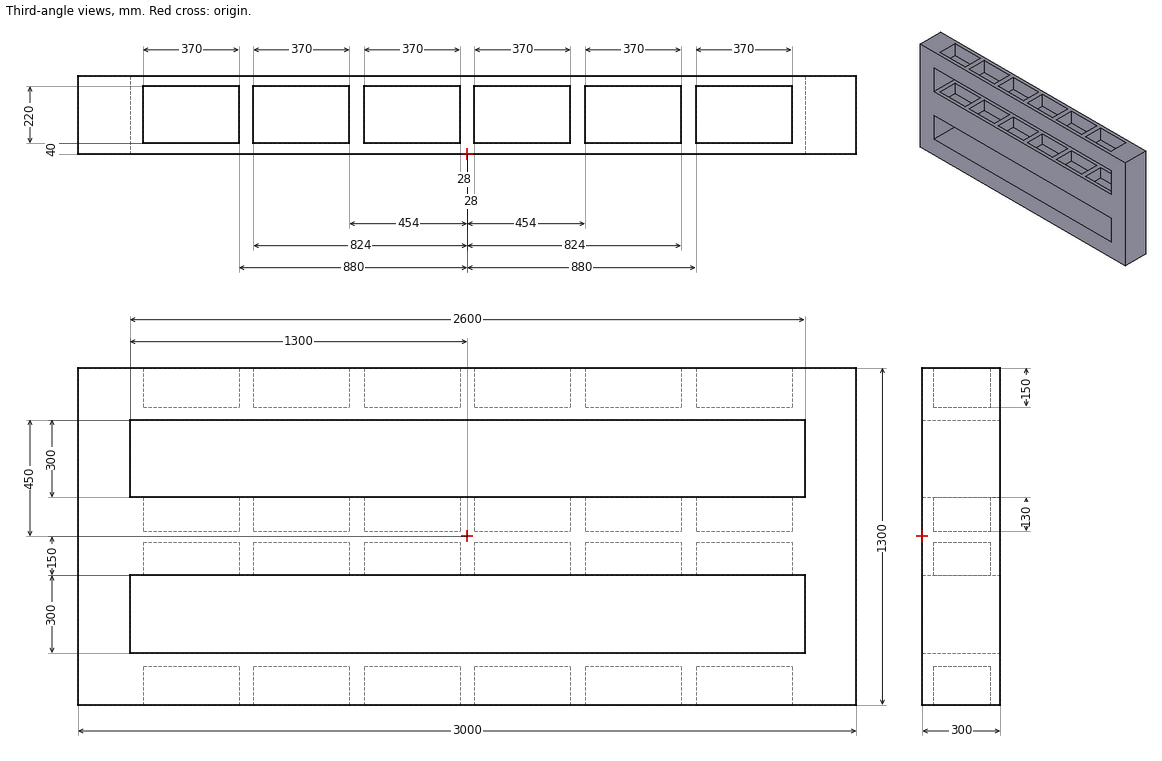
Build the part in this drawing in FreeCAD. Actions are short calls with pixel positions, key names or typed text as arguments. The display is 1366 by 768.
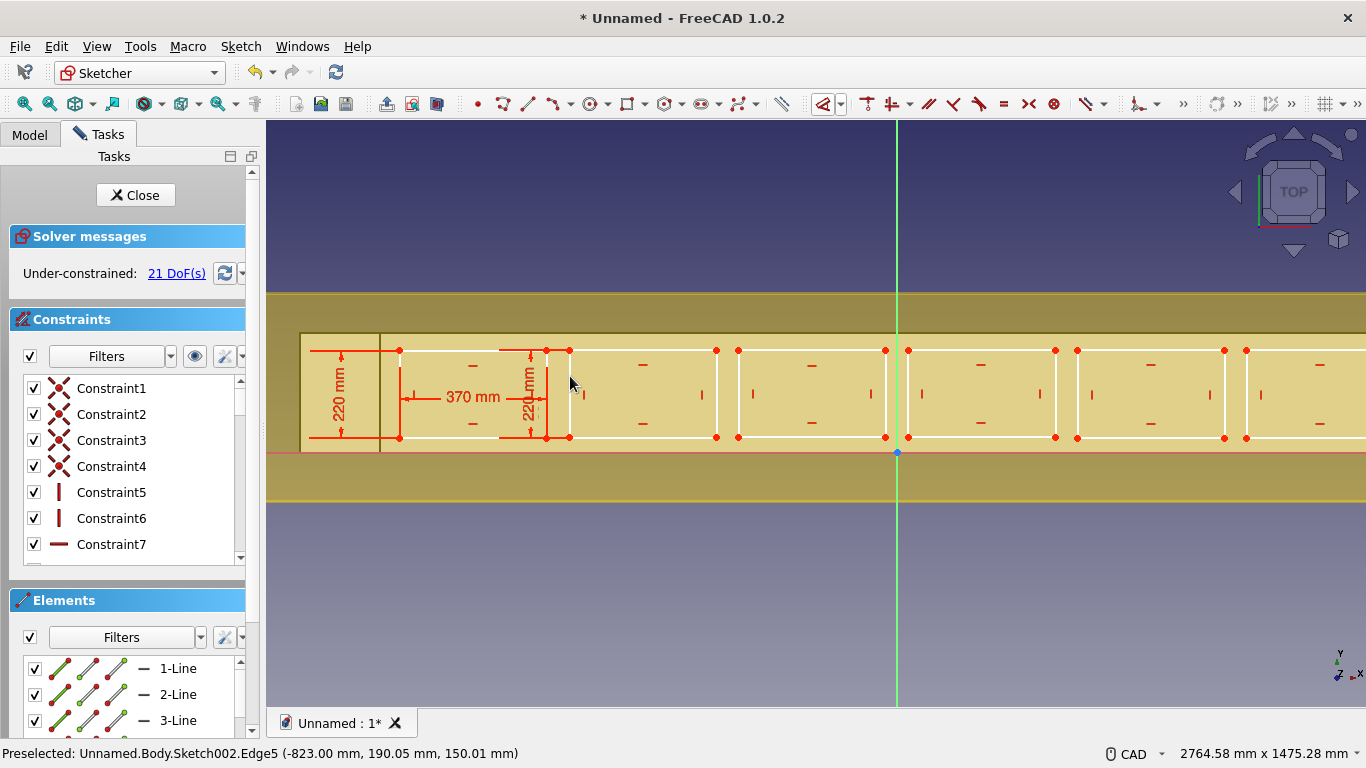
click(614, 438)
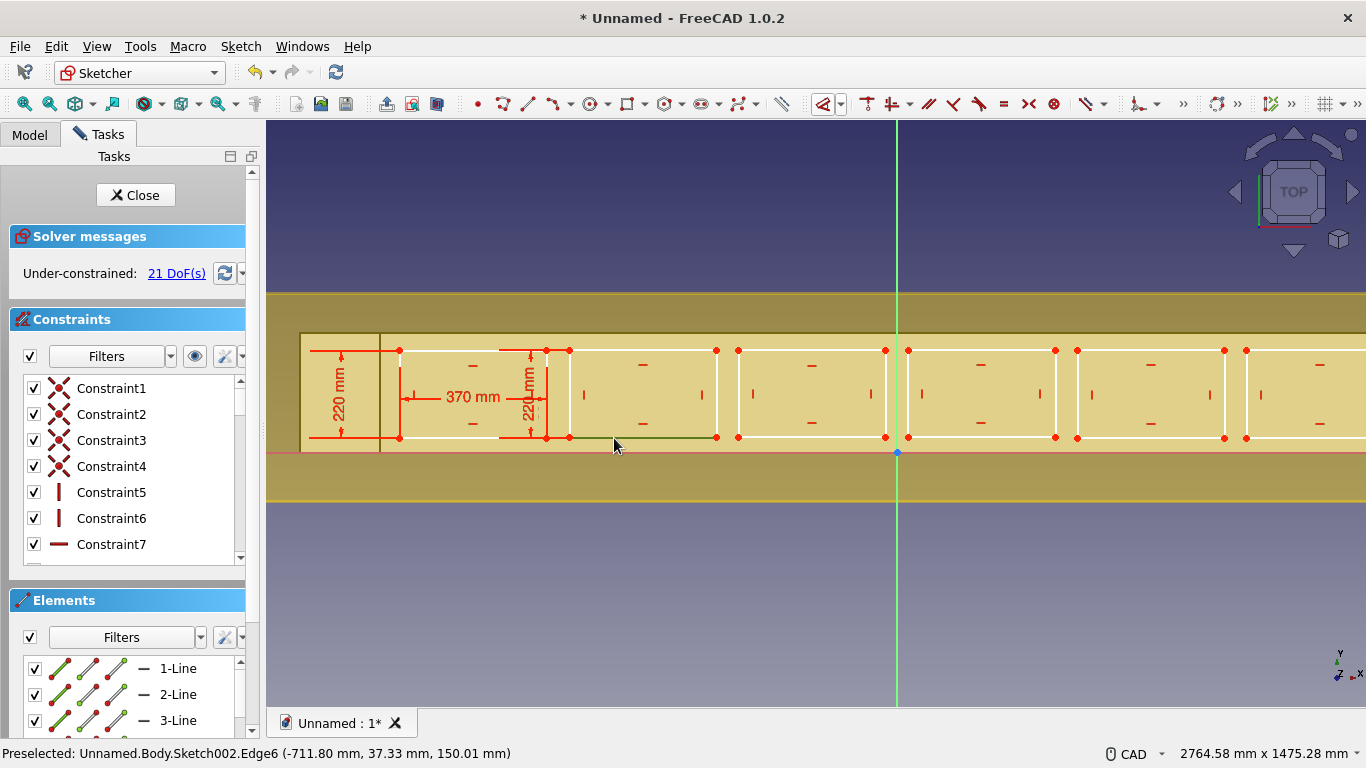
key(l)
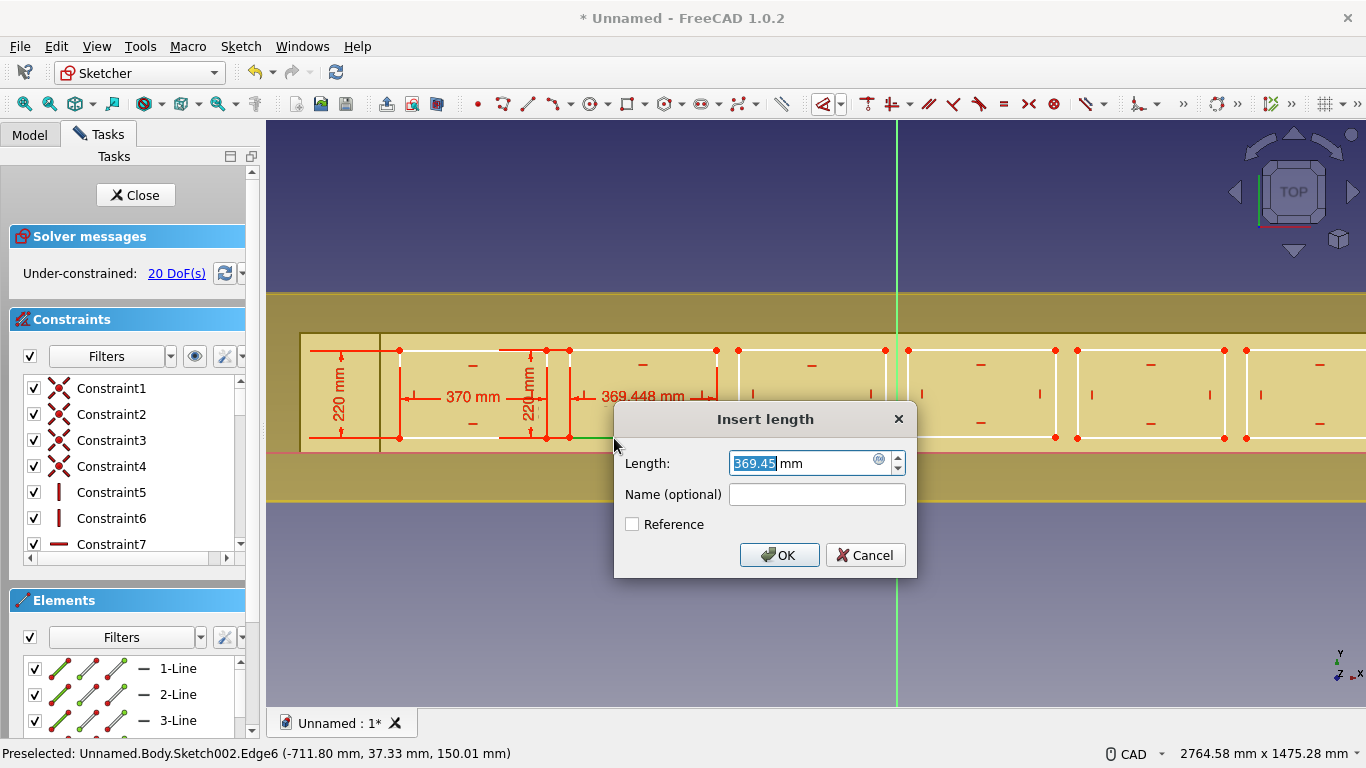
text(370)
key(Return)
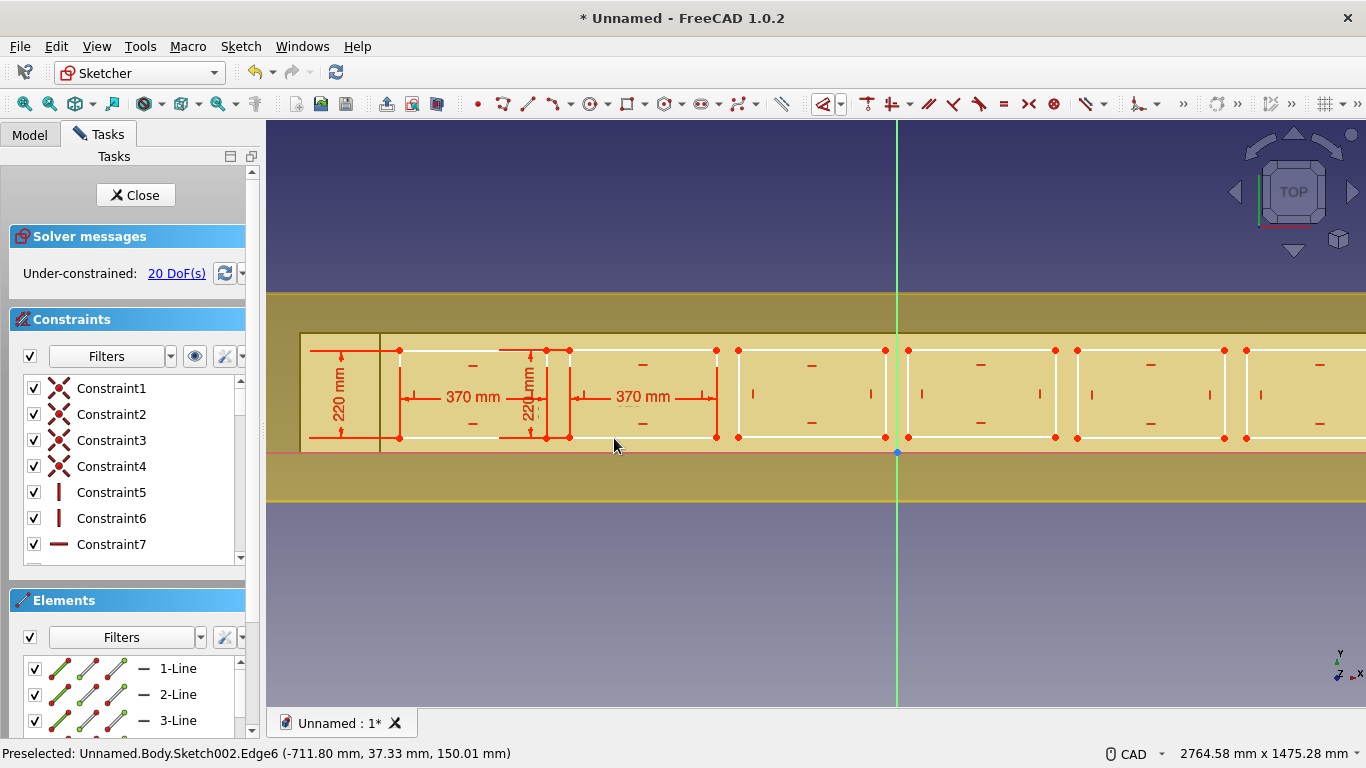
click(739, 376)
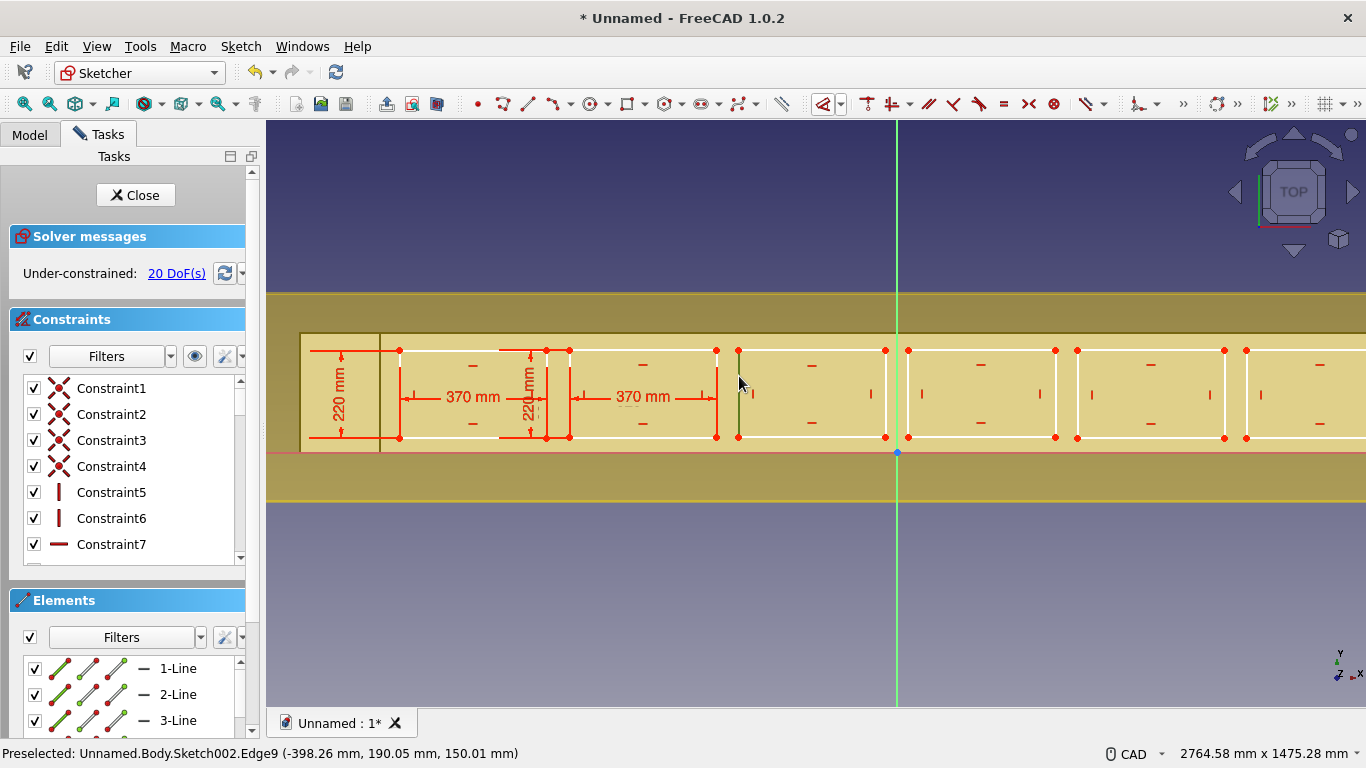
key(i)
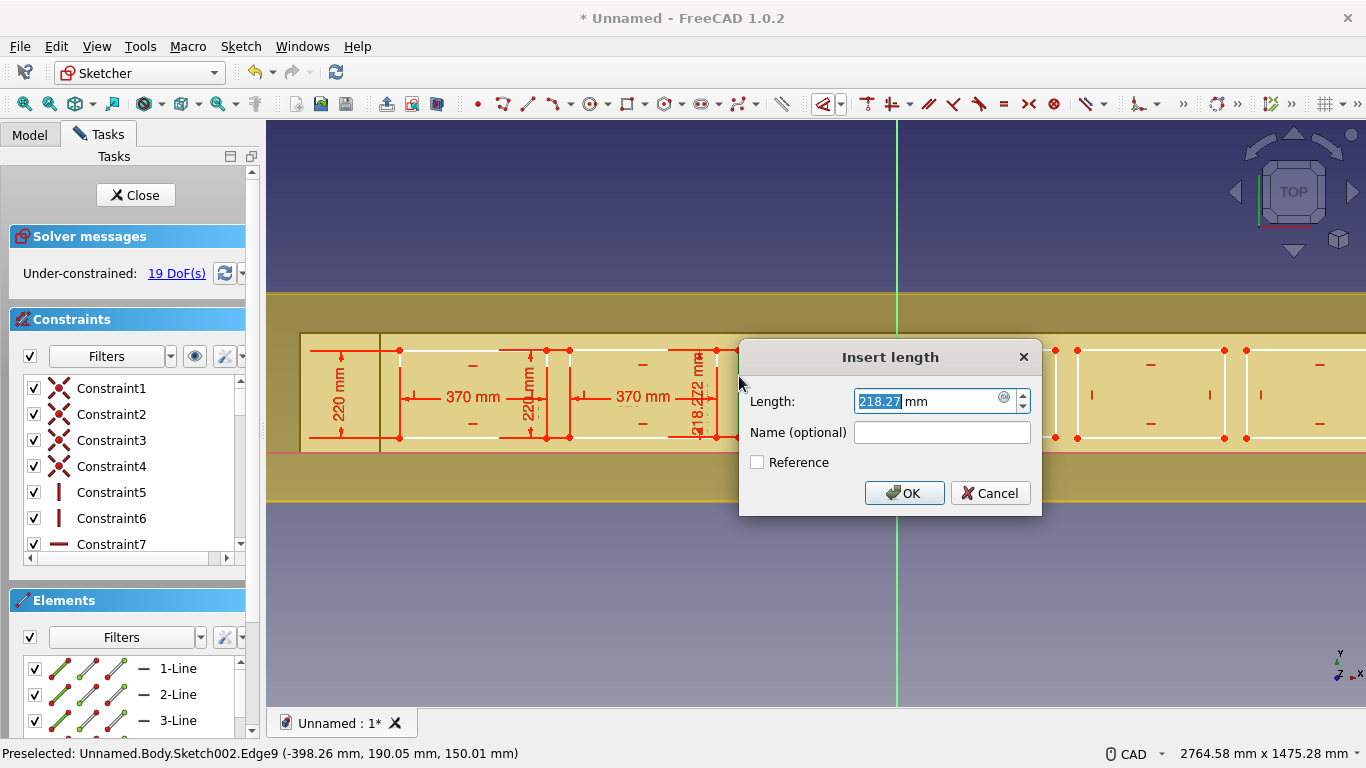
text(220)
key(Return)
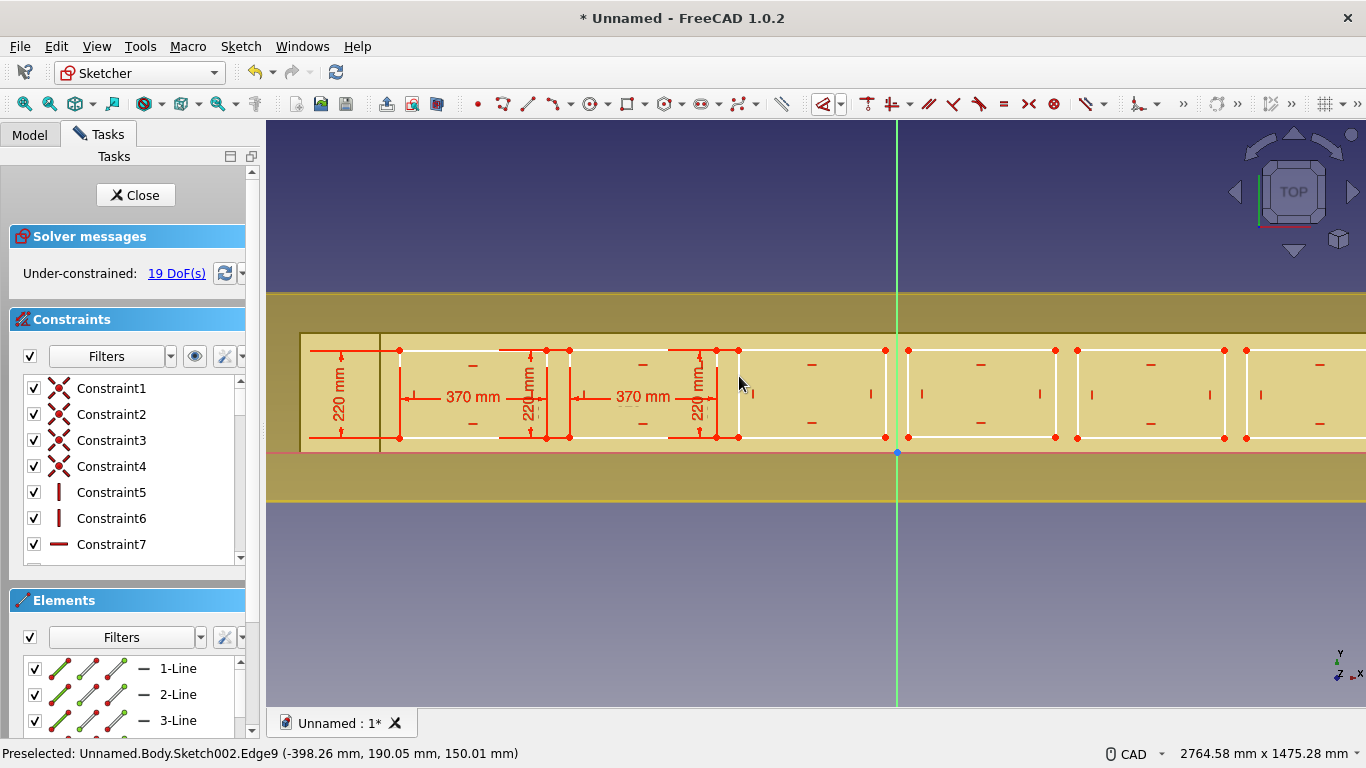
click(783, 438)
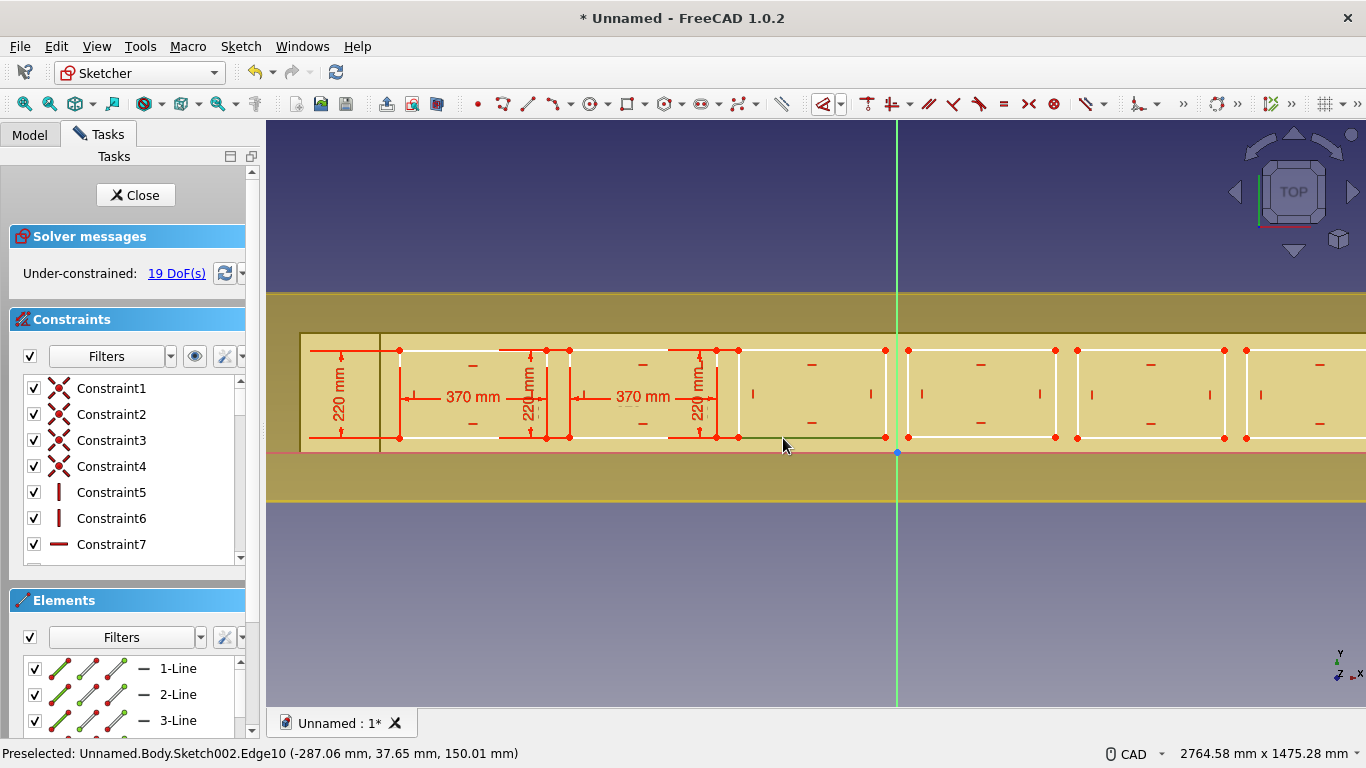
key(l)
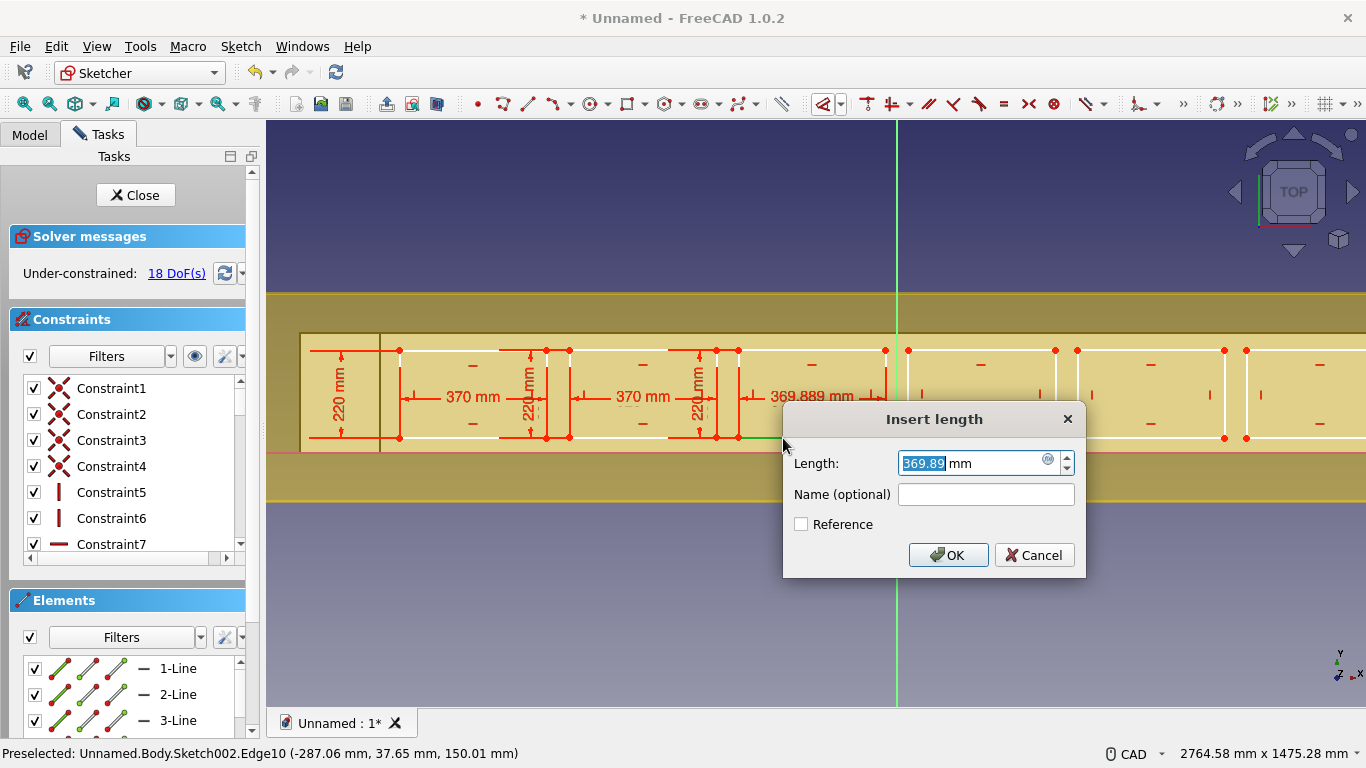
text(370)
key(Return)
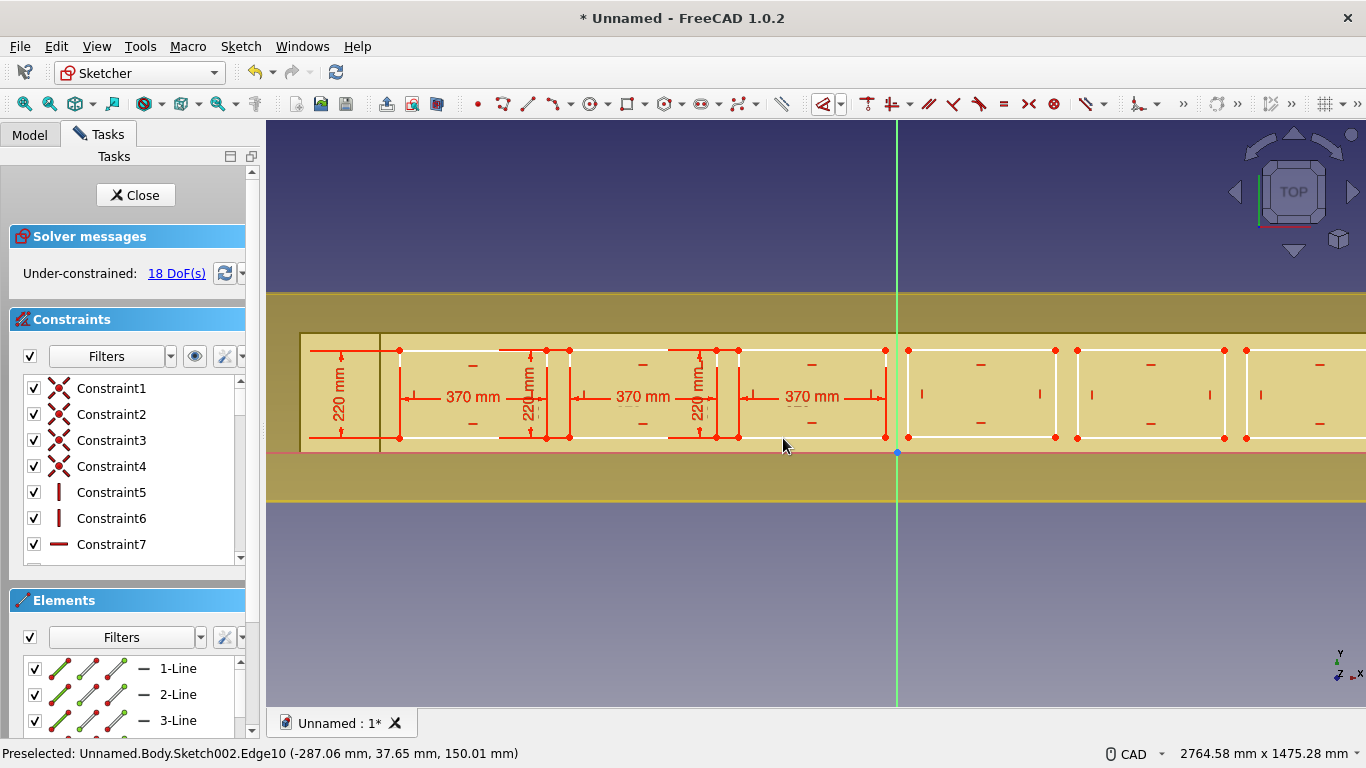
scroll(908, 376, up, 2)